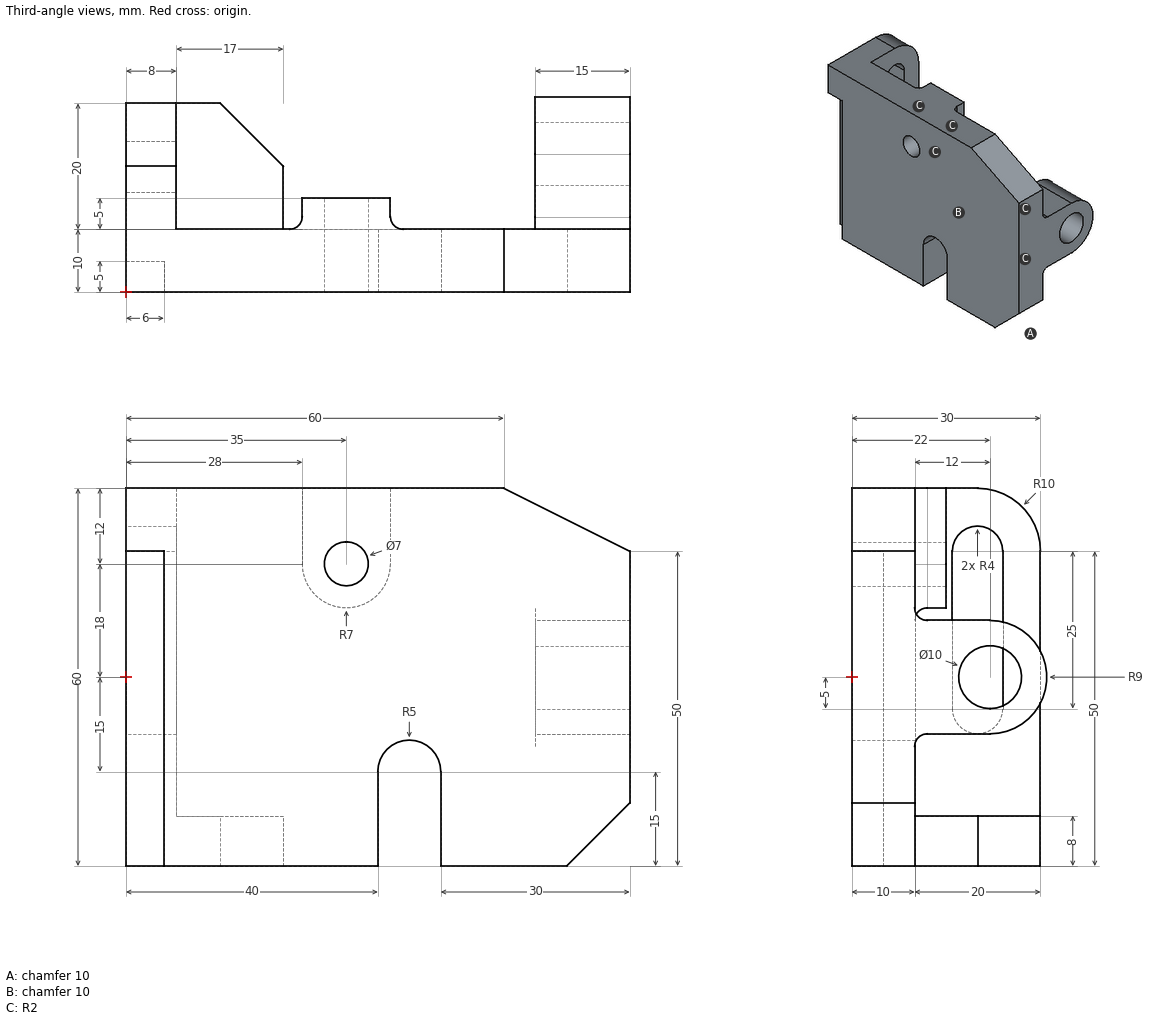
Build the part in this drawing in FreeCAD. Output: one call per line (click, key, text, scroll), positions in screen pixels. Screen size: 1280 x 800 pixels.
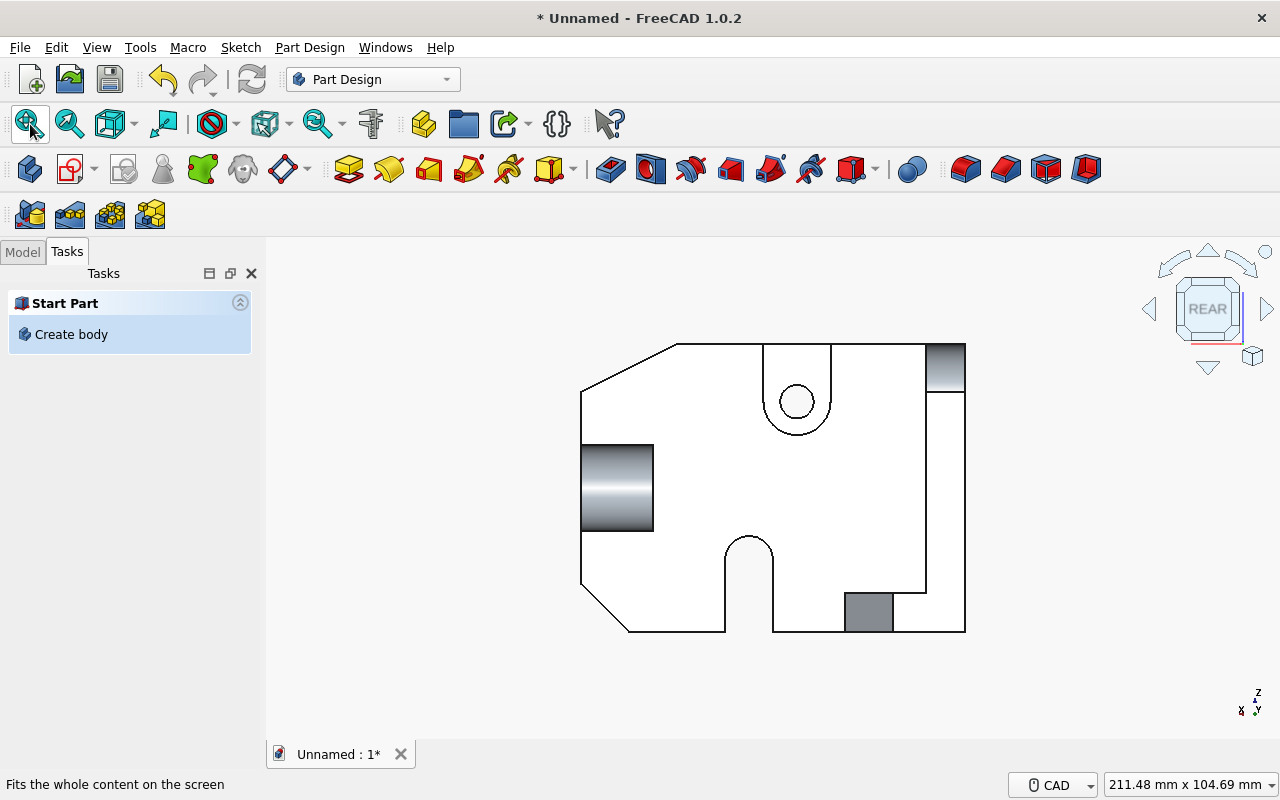
key(6)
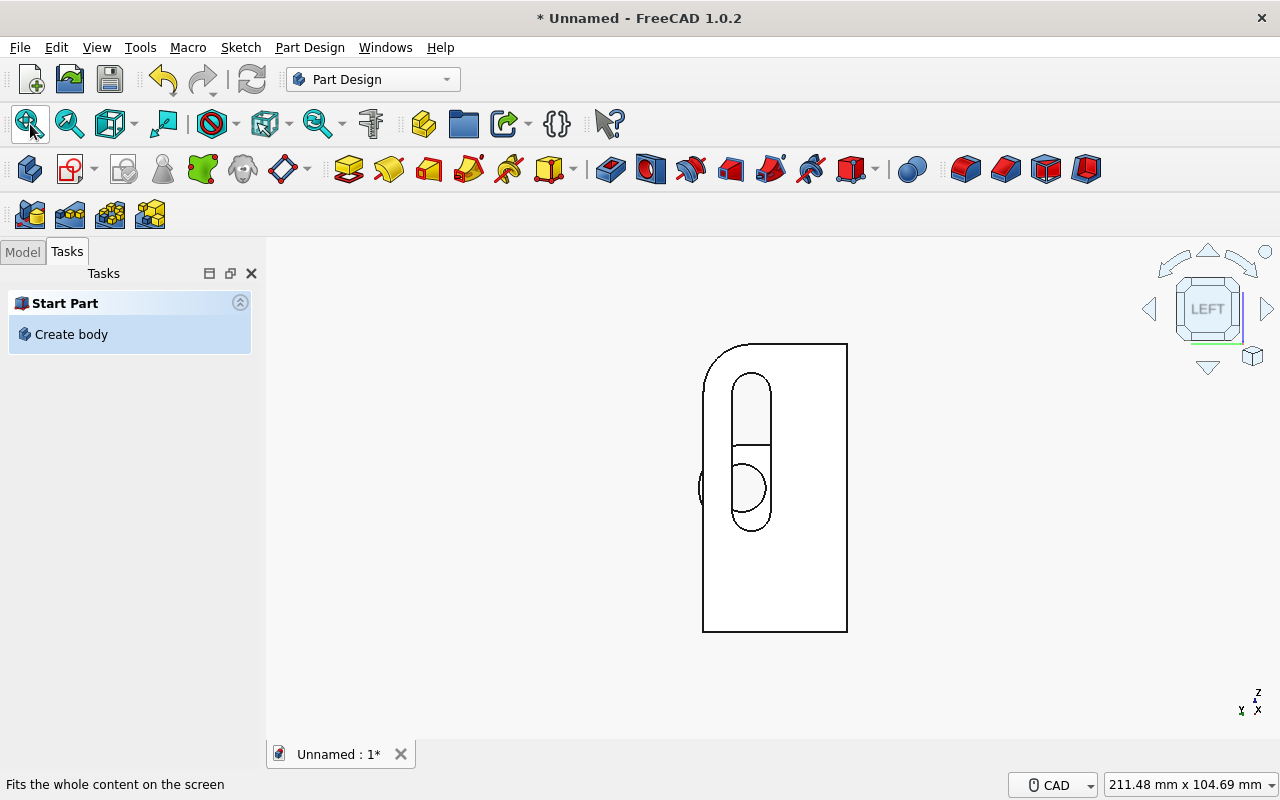
key(v)
key(3)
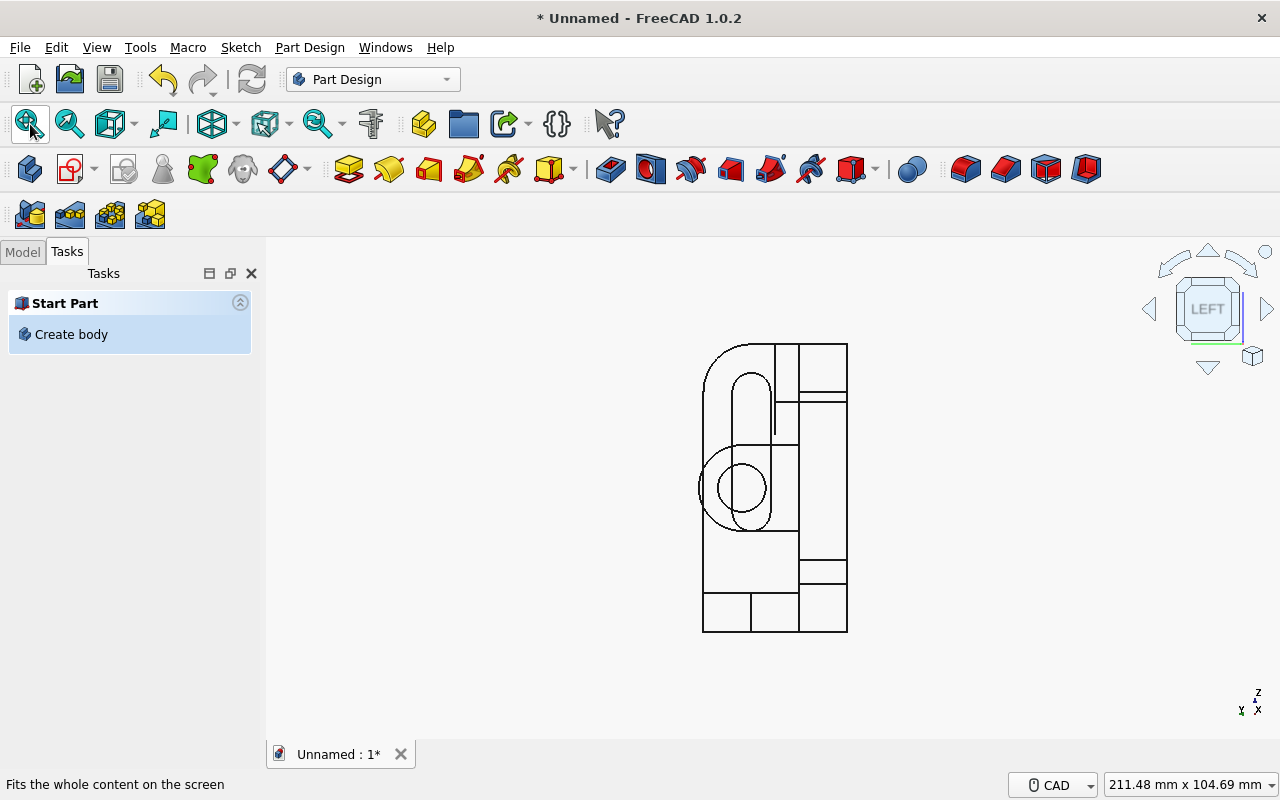
key(0)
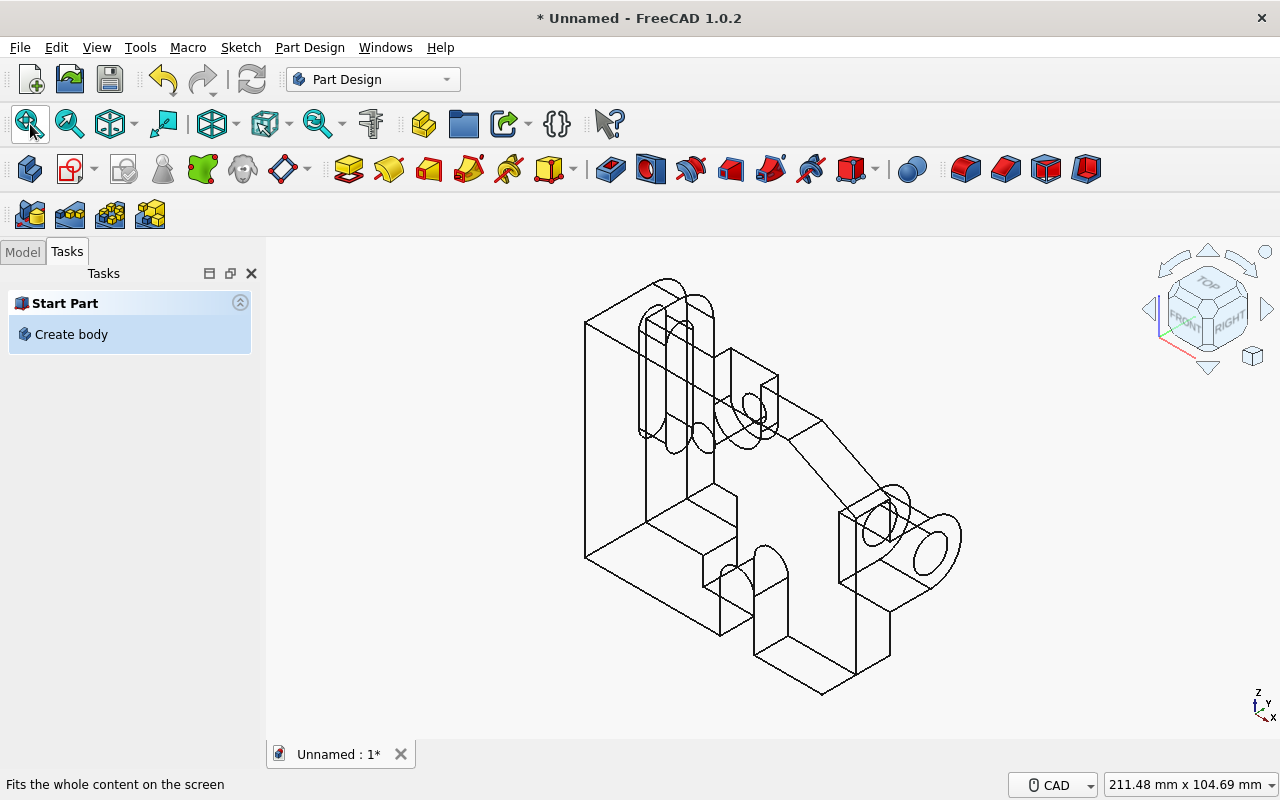
click(865, 597)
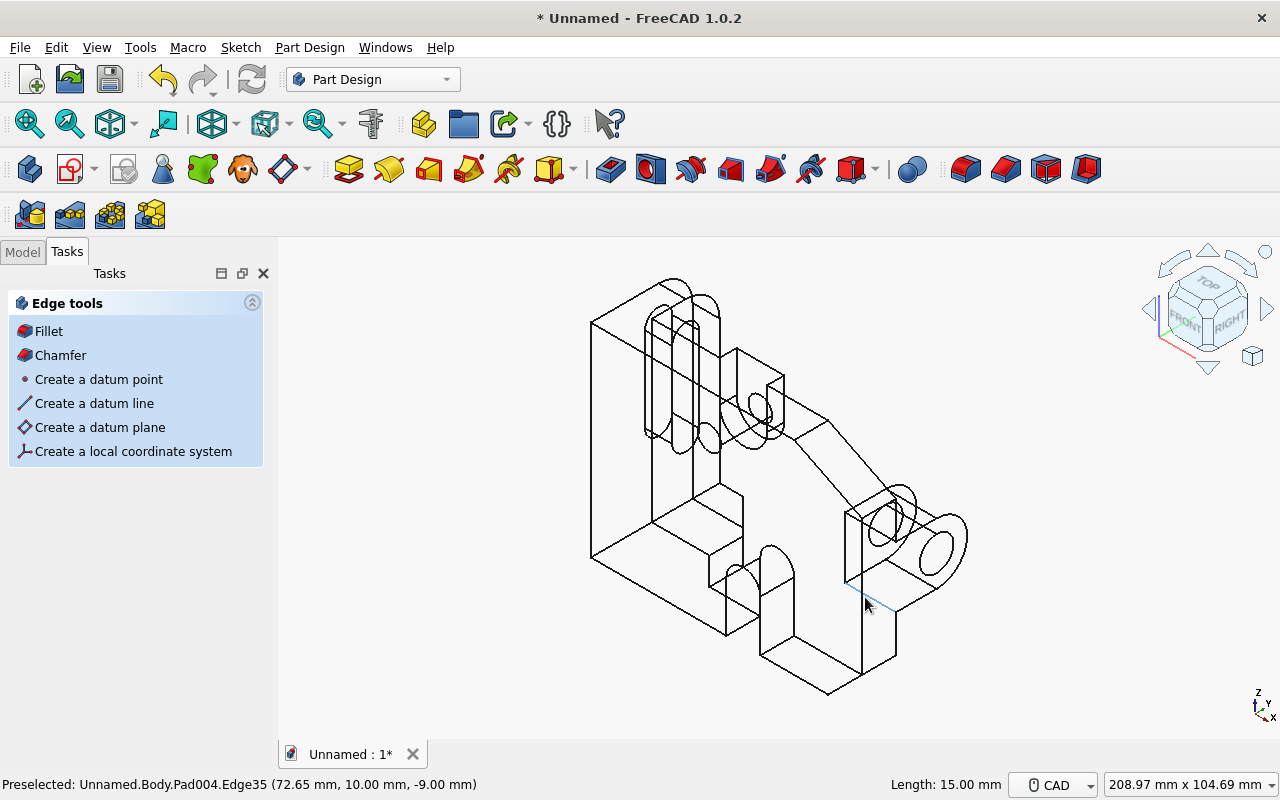
click(871, 526, ctrl)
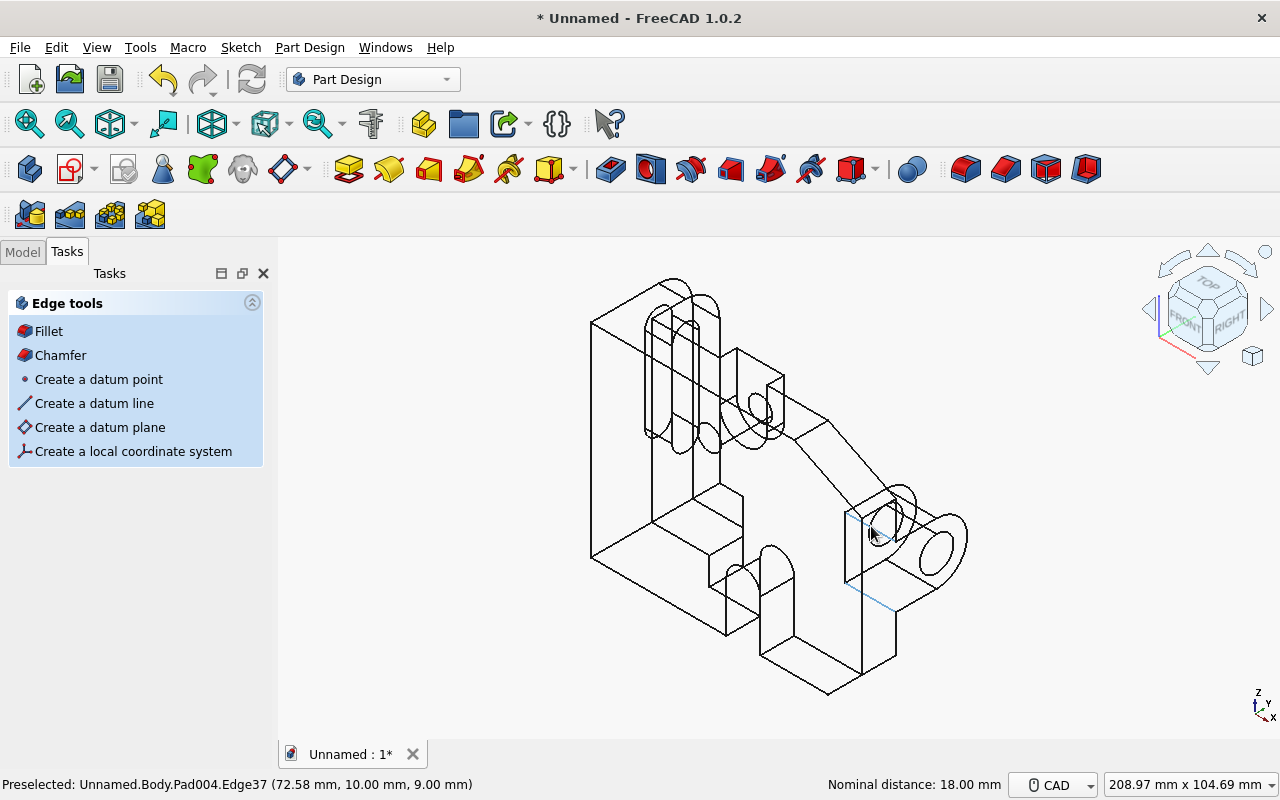
click(743, 445, ctrl)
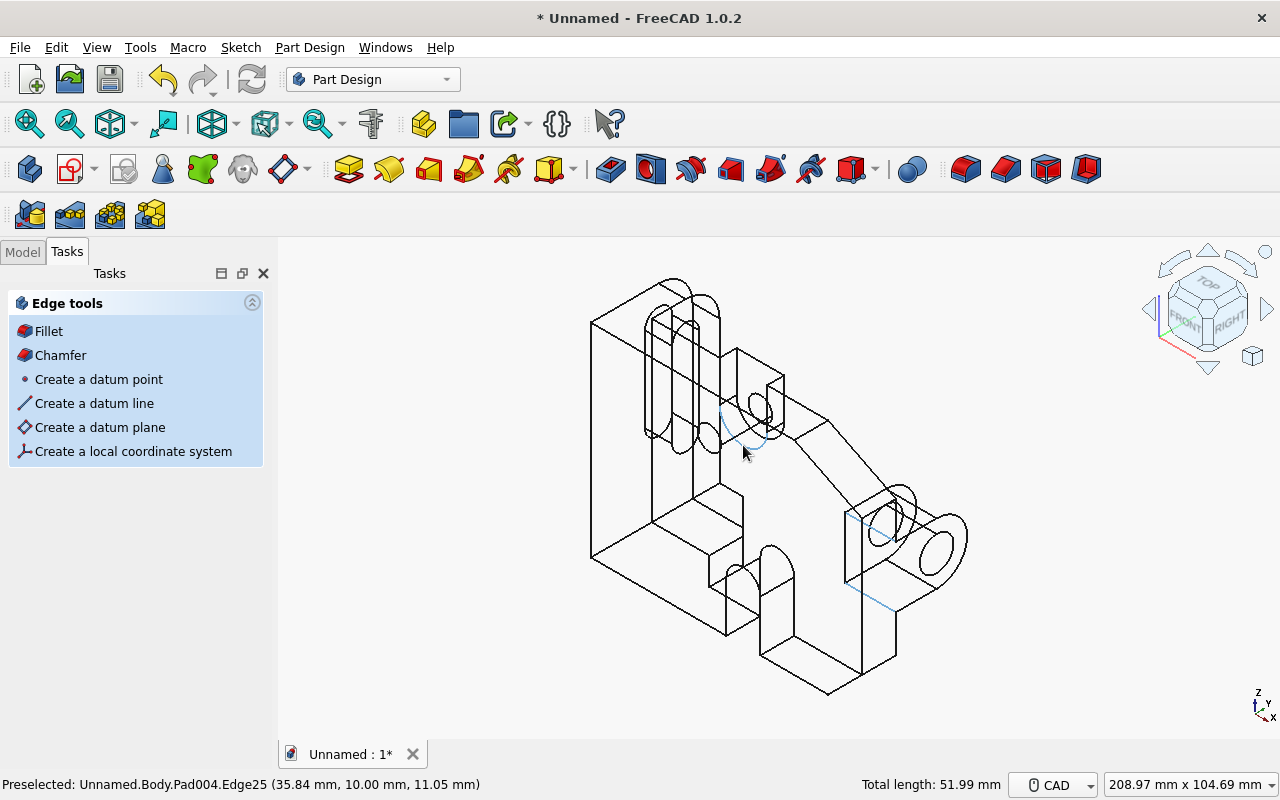
click(720, 380, ctrl)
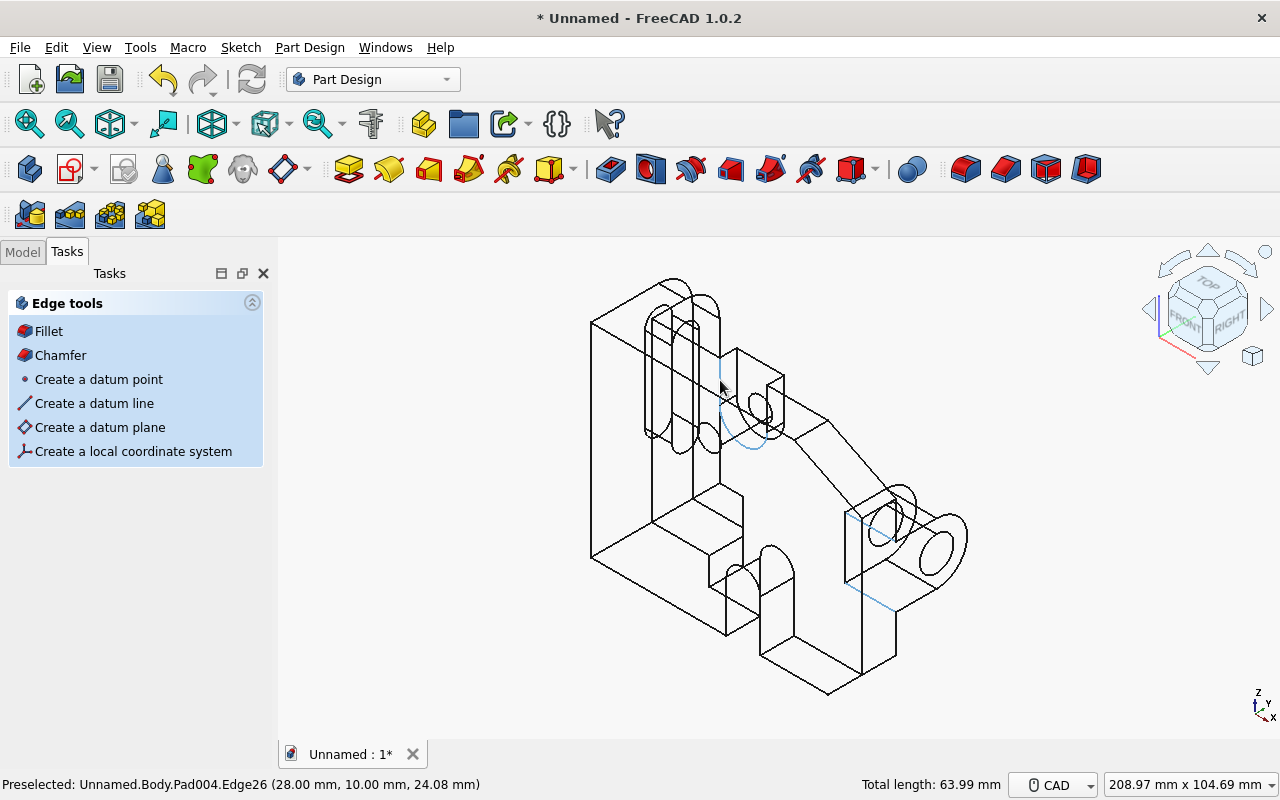
click(767, 408, ctrl)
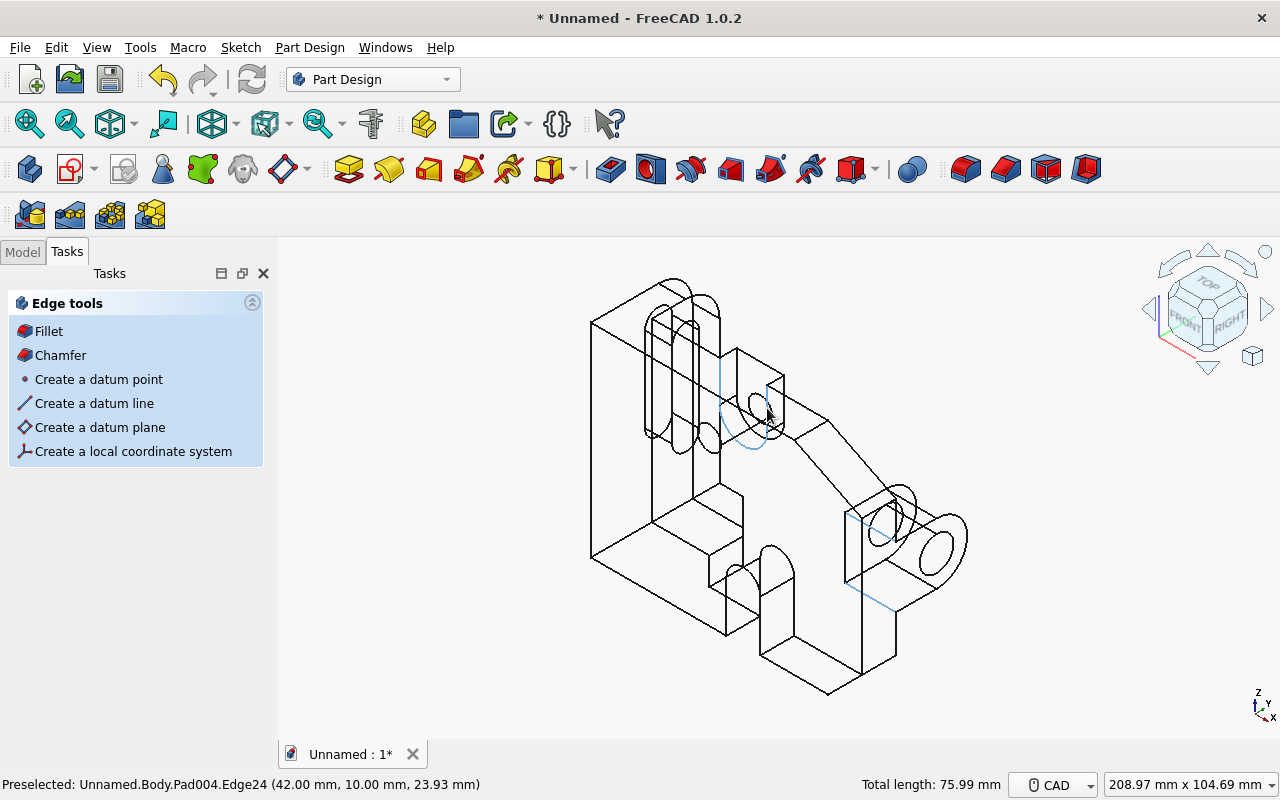
key(v)
key(1)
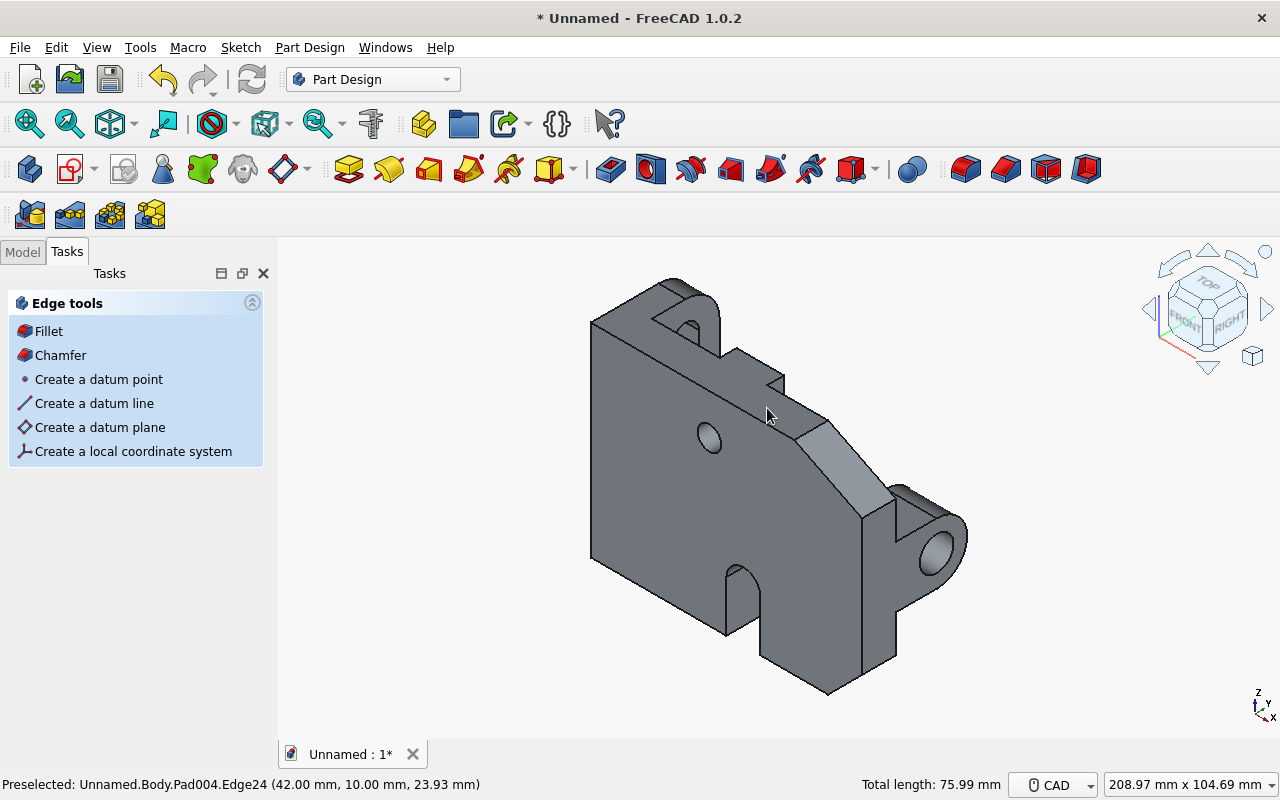
click(966, 170)